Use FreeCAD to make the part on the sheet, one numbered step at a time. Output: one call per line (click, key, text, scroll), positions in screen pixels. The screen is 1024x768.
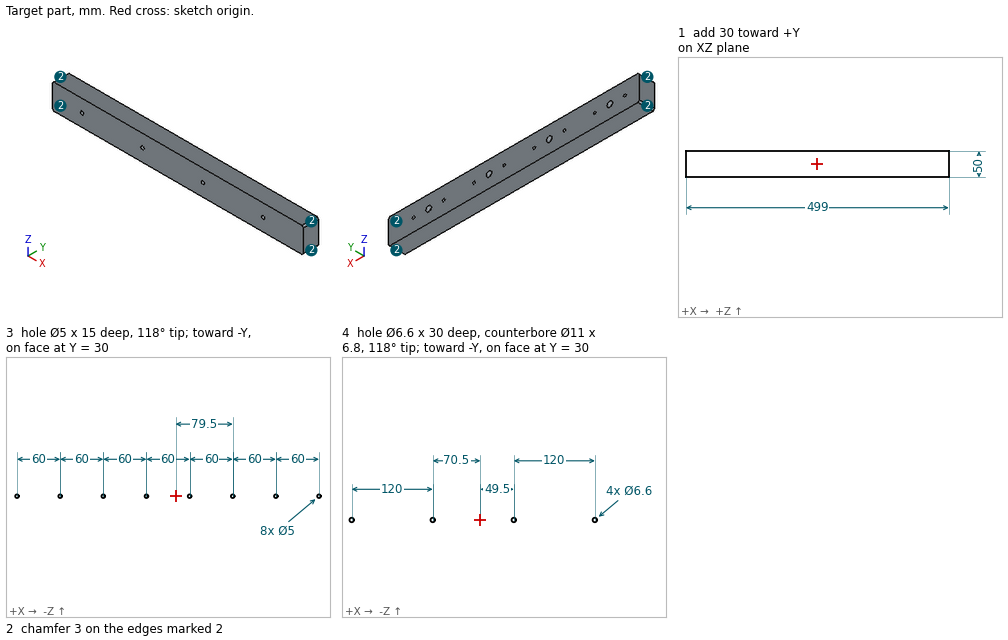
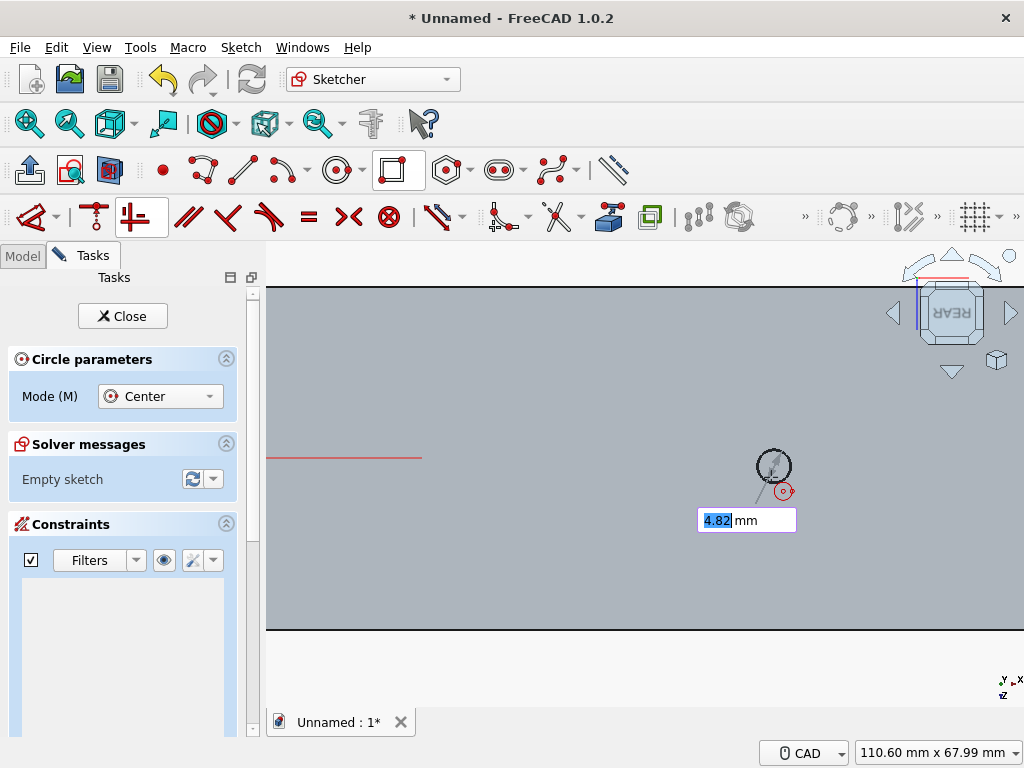
click(767, 474)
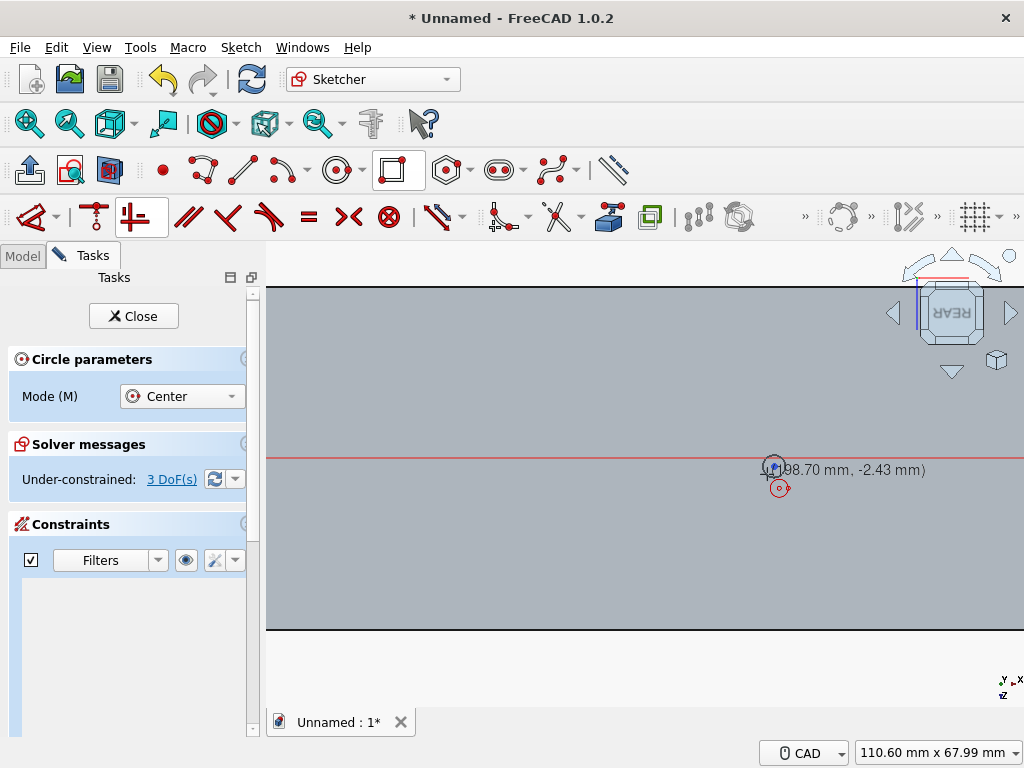
scroll(361, 458, up, 2)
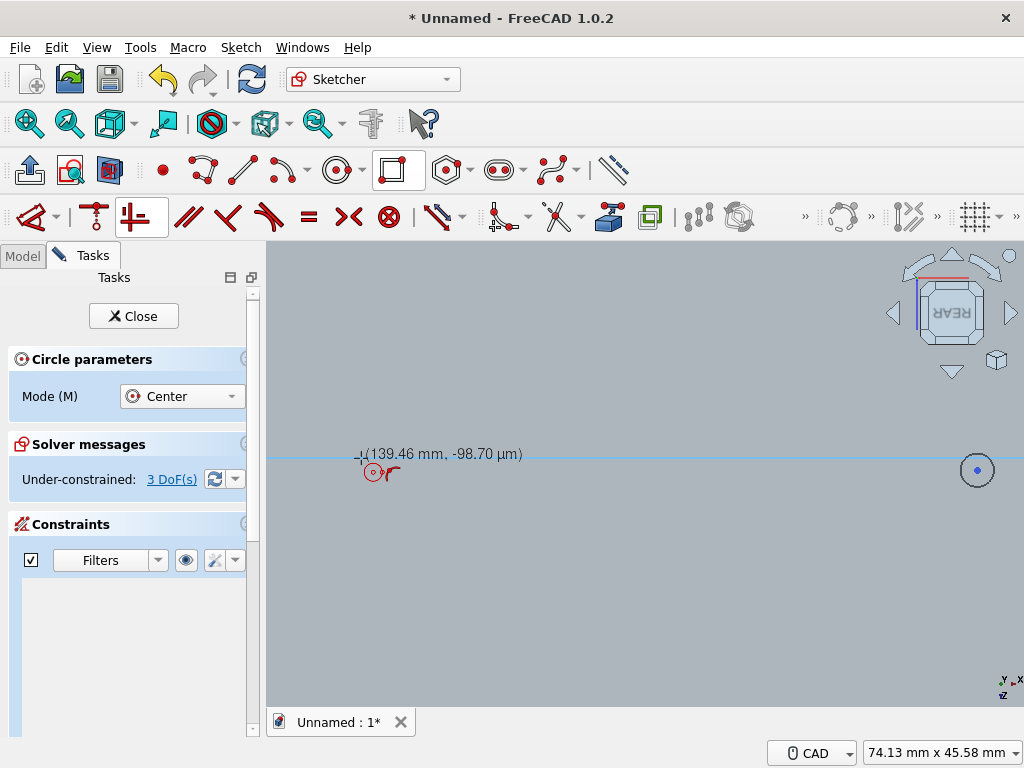
scroll(751, 476, down, 12)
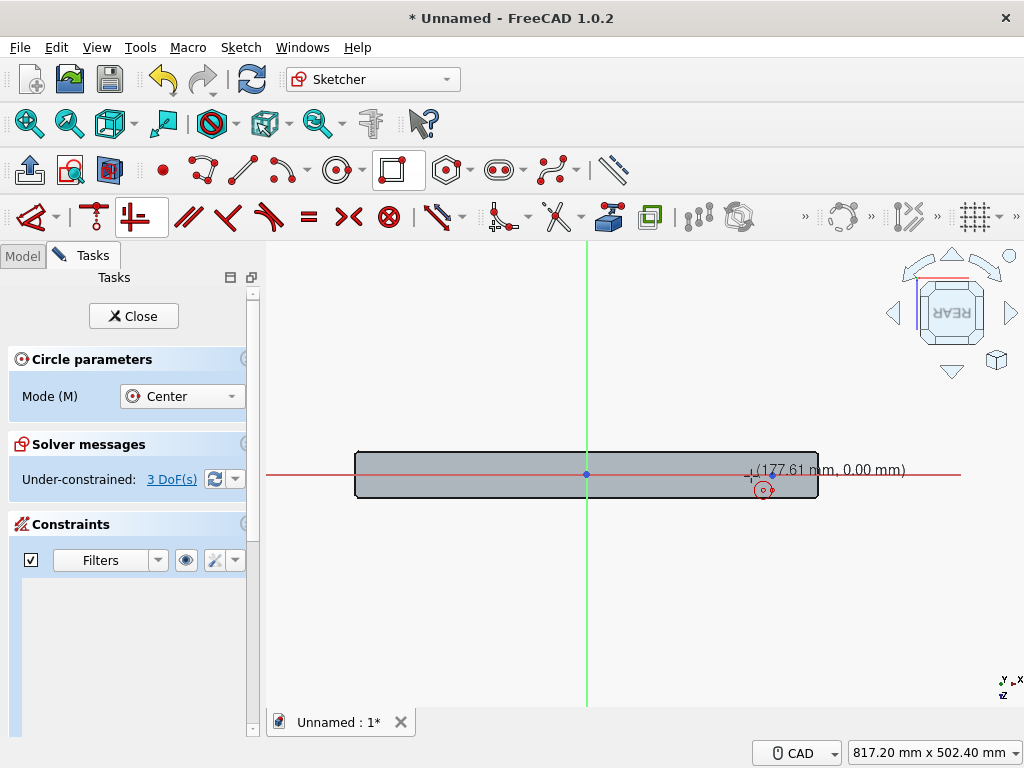
click(716, 475)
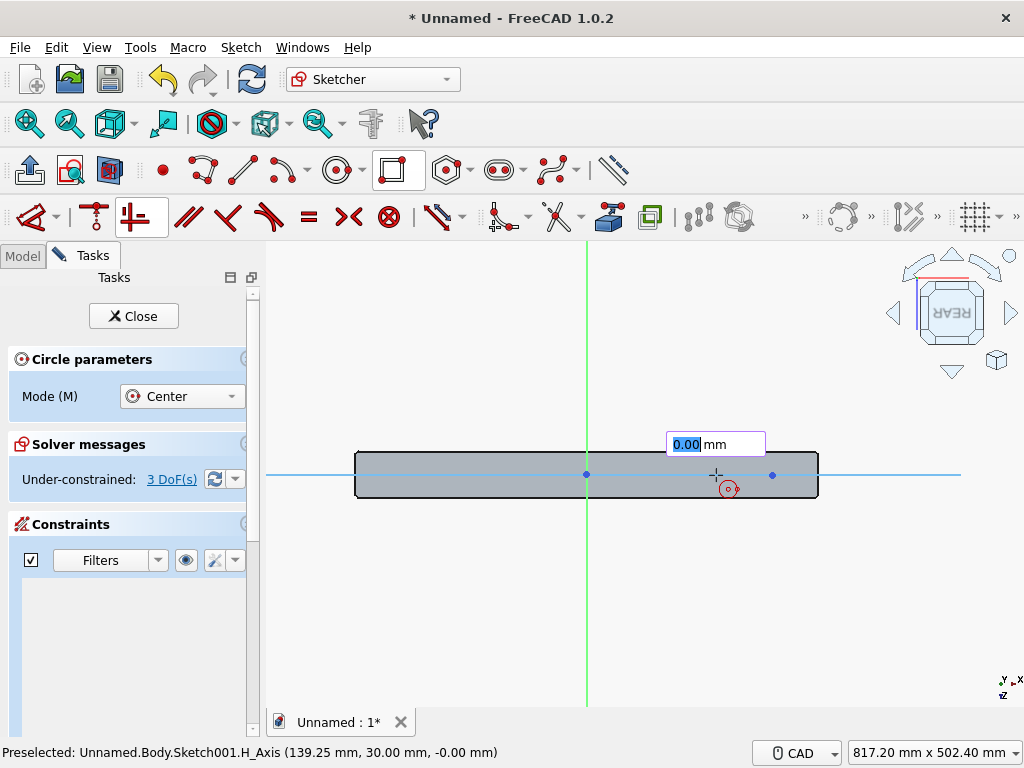
scroll(715, 477, up, 10)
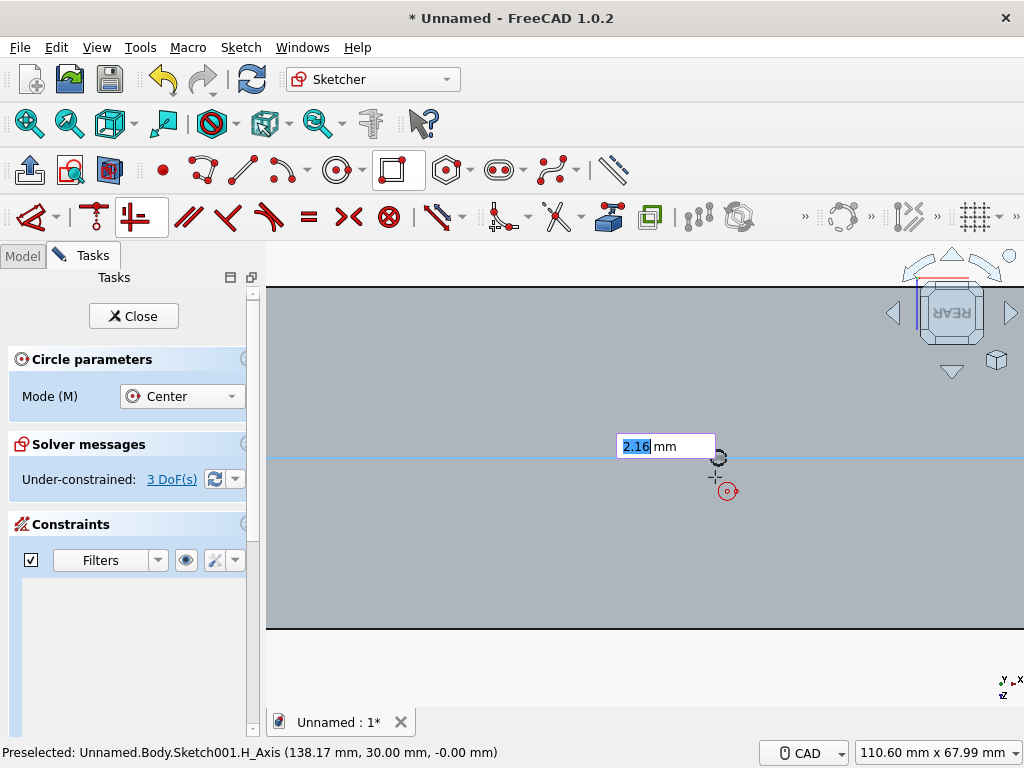
click(714, 474)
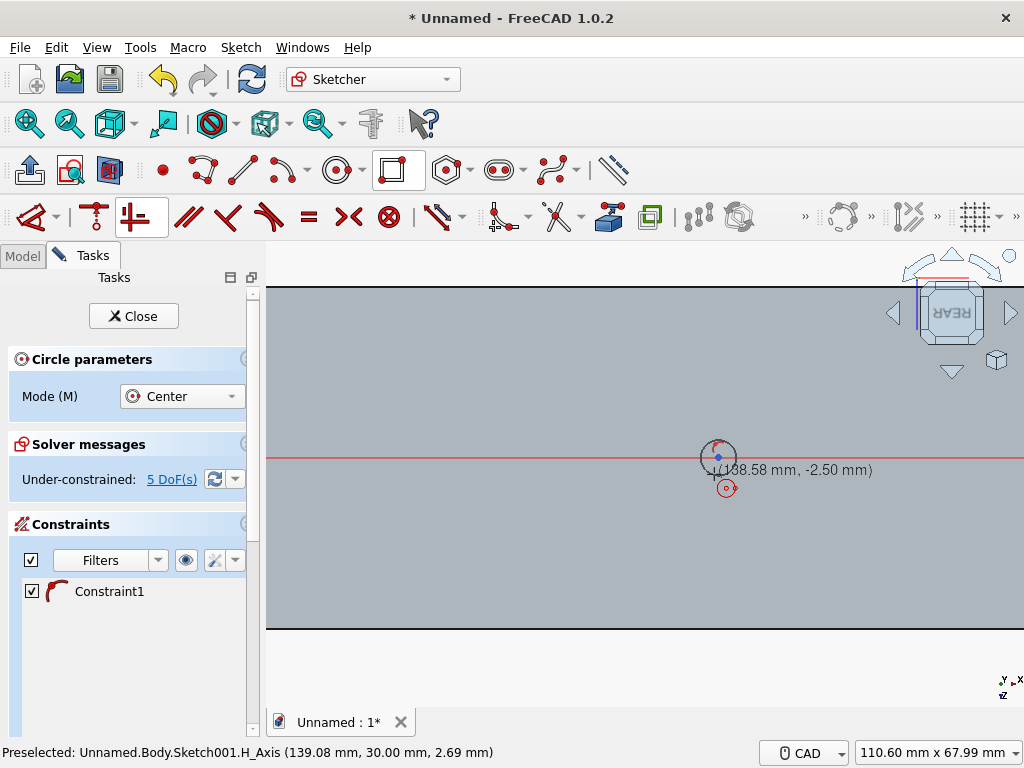
scroll(309, 458, up, 2)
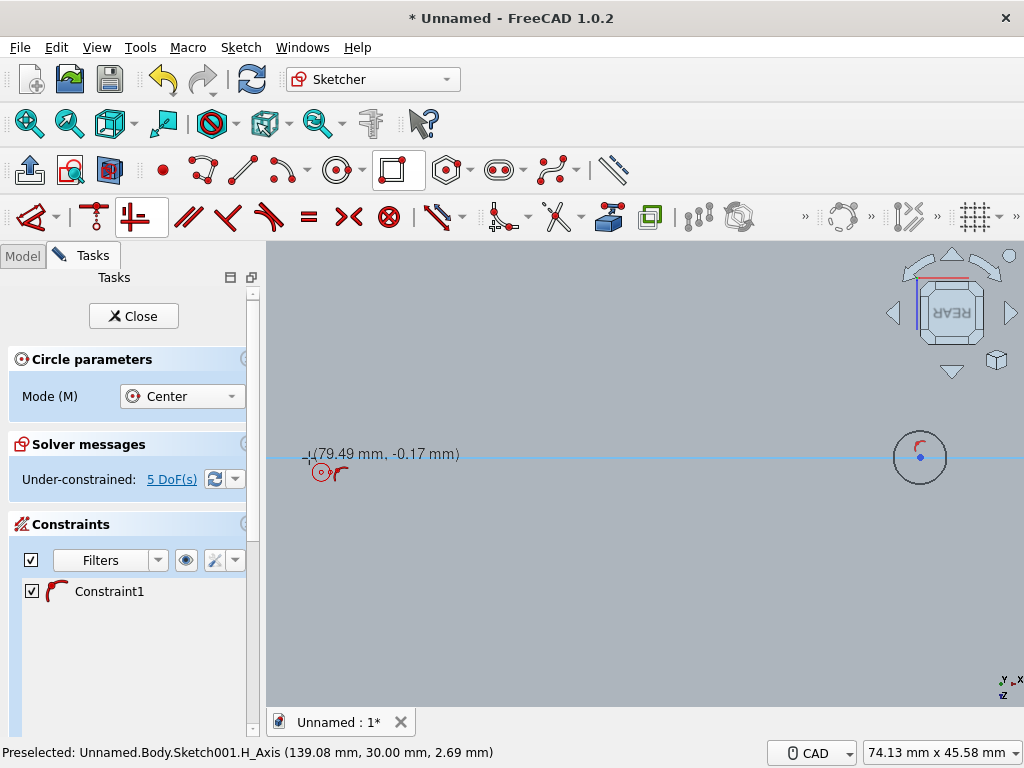
scroll(695, 476, down, 12)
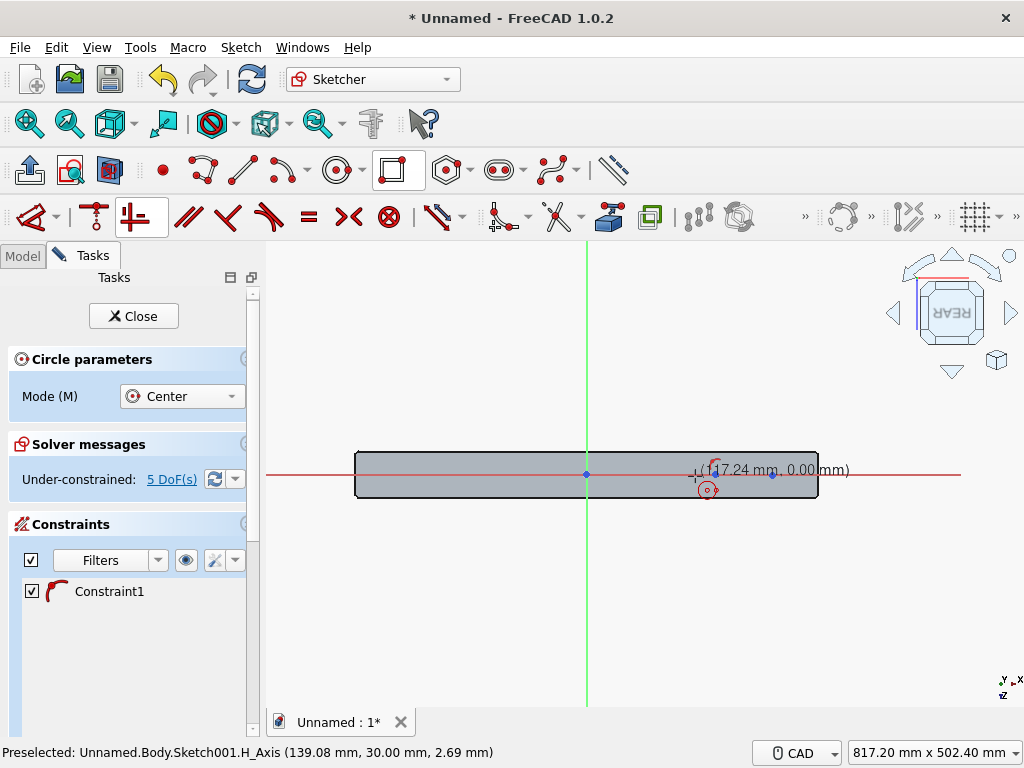
click(661, 475)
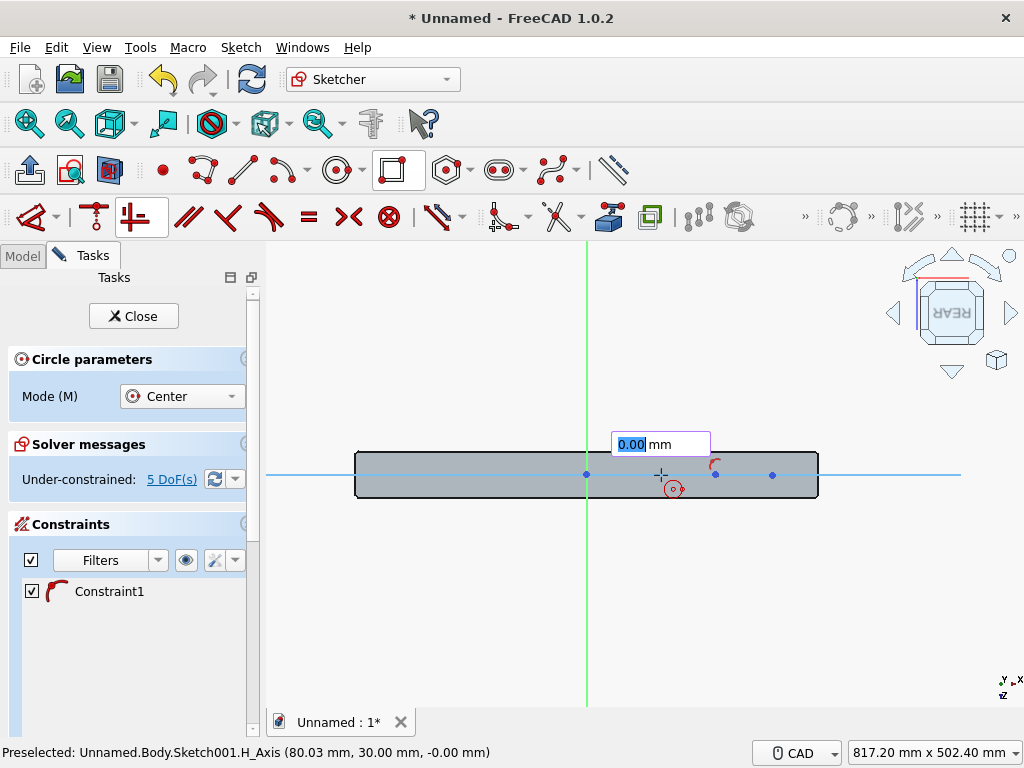
scroll(660, 477, up, 10)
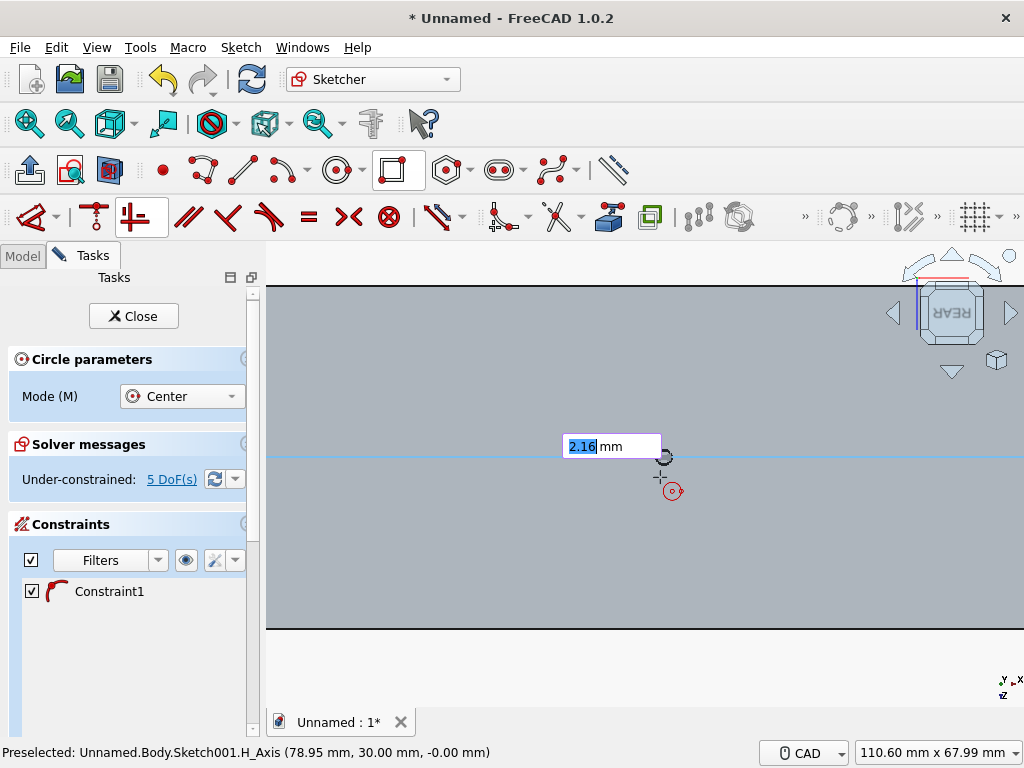
click(655, 474)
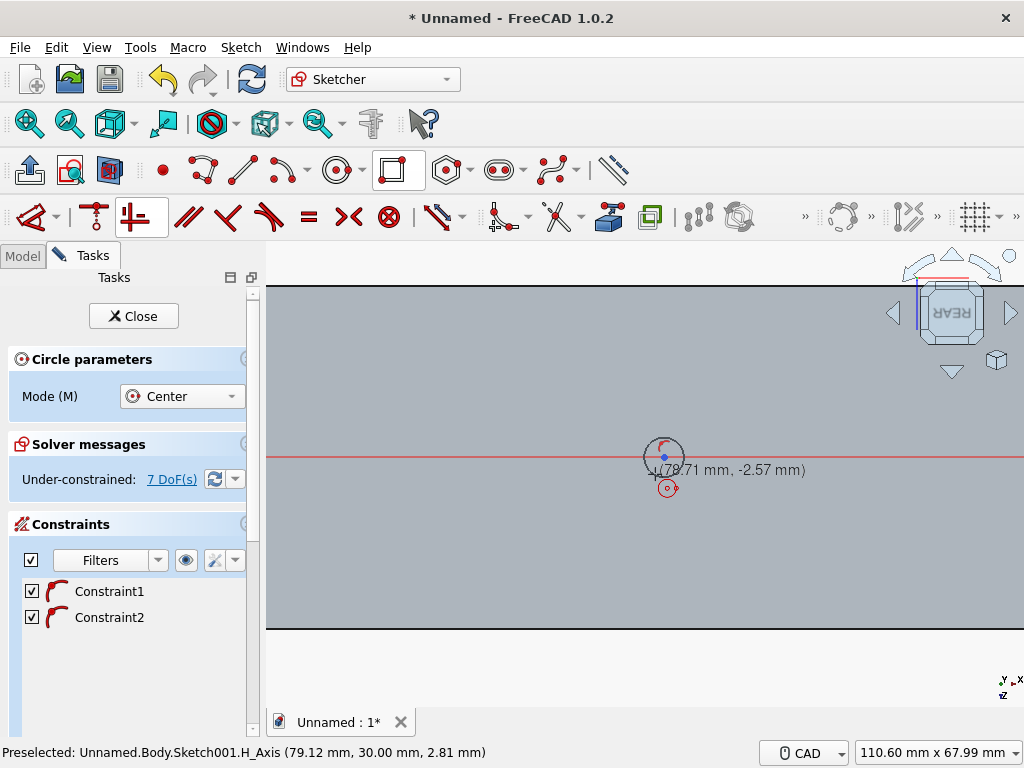
scroll(660, 477, down, 10)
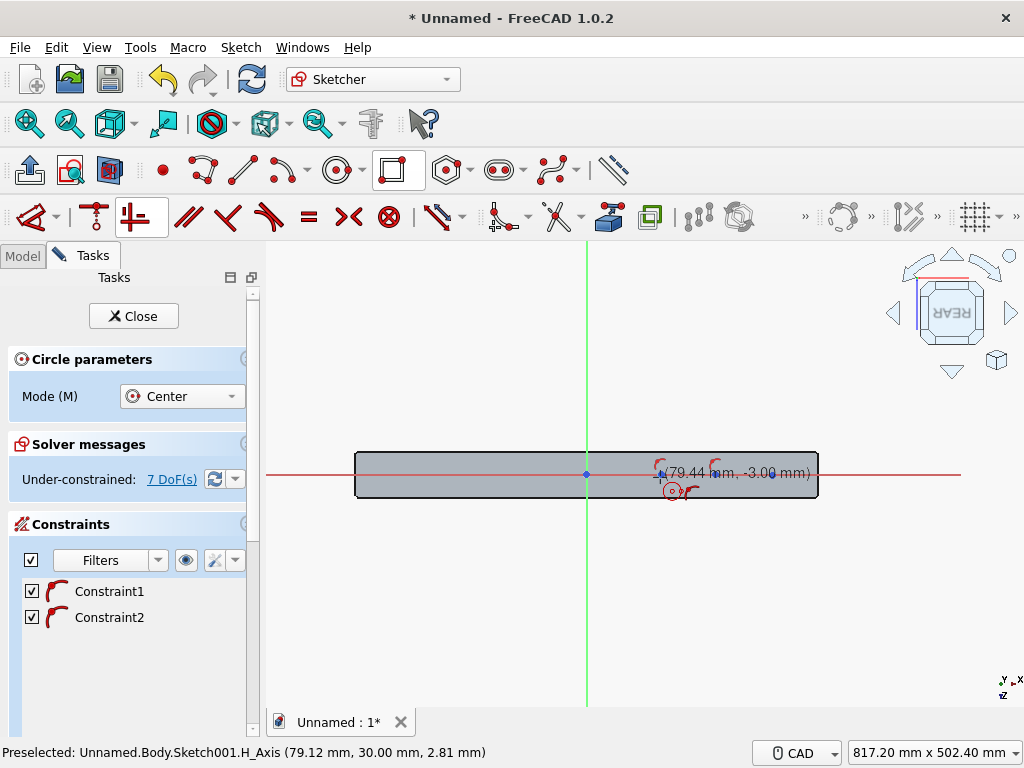
scroll(605, 475, up, 12)